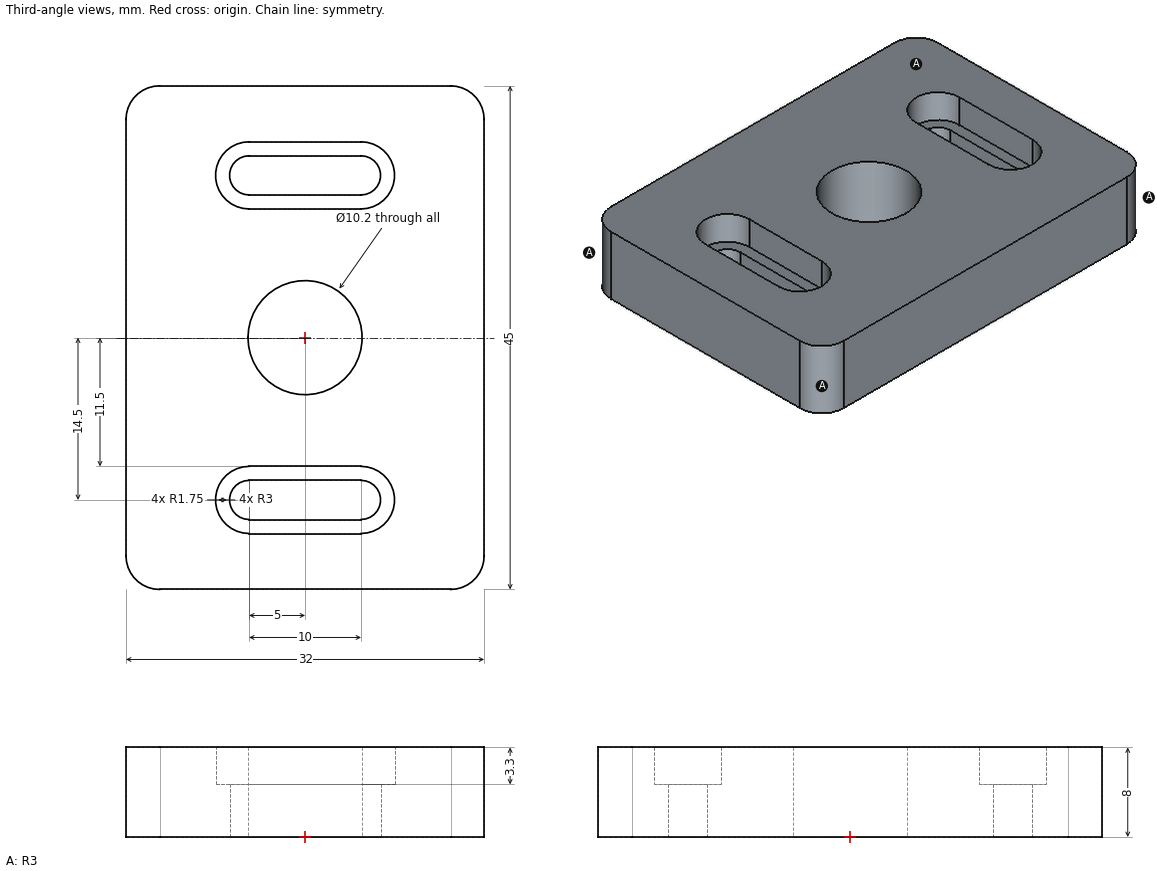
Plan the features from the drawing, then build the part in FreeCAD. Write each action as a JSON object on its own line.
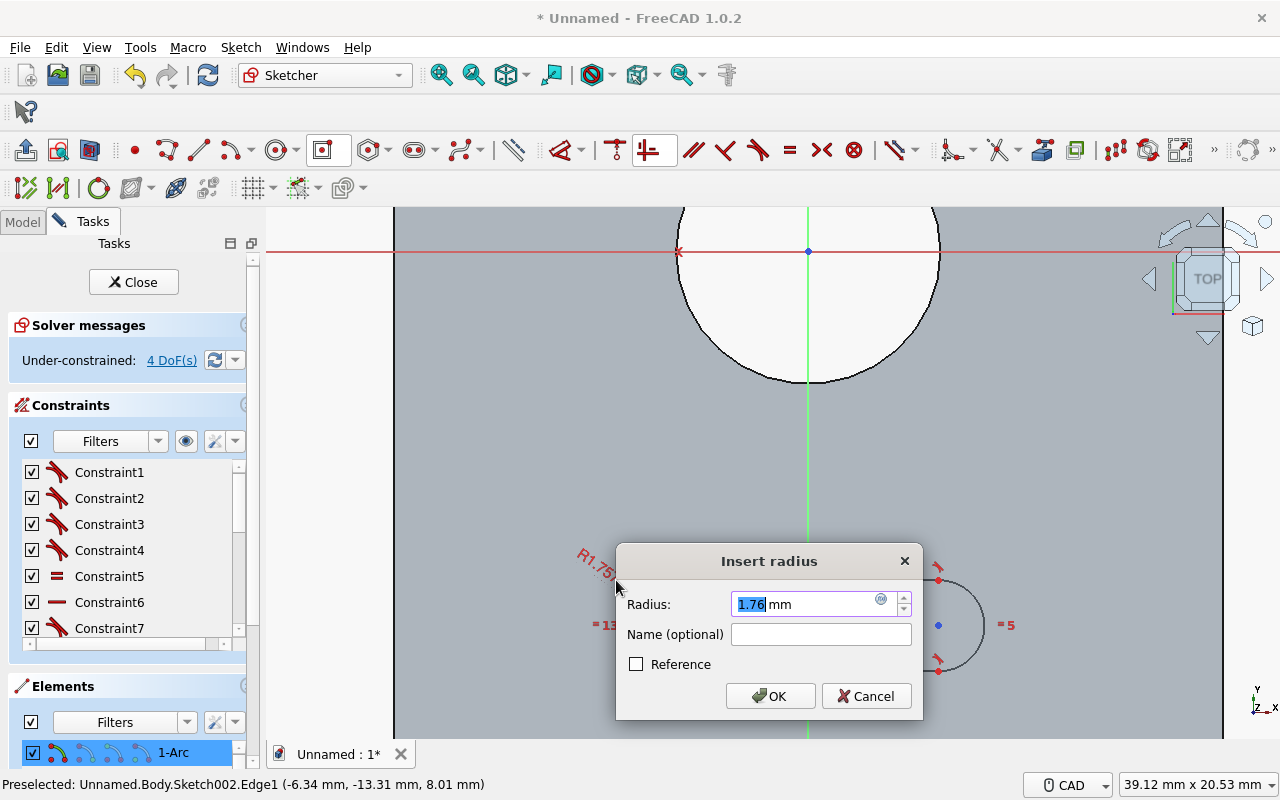
{"action": "type", "text": "1.75"}
{"action": "key", "text": "Return"}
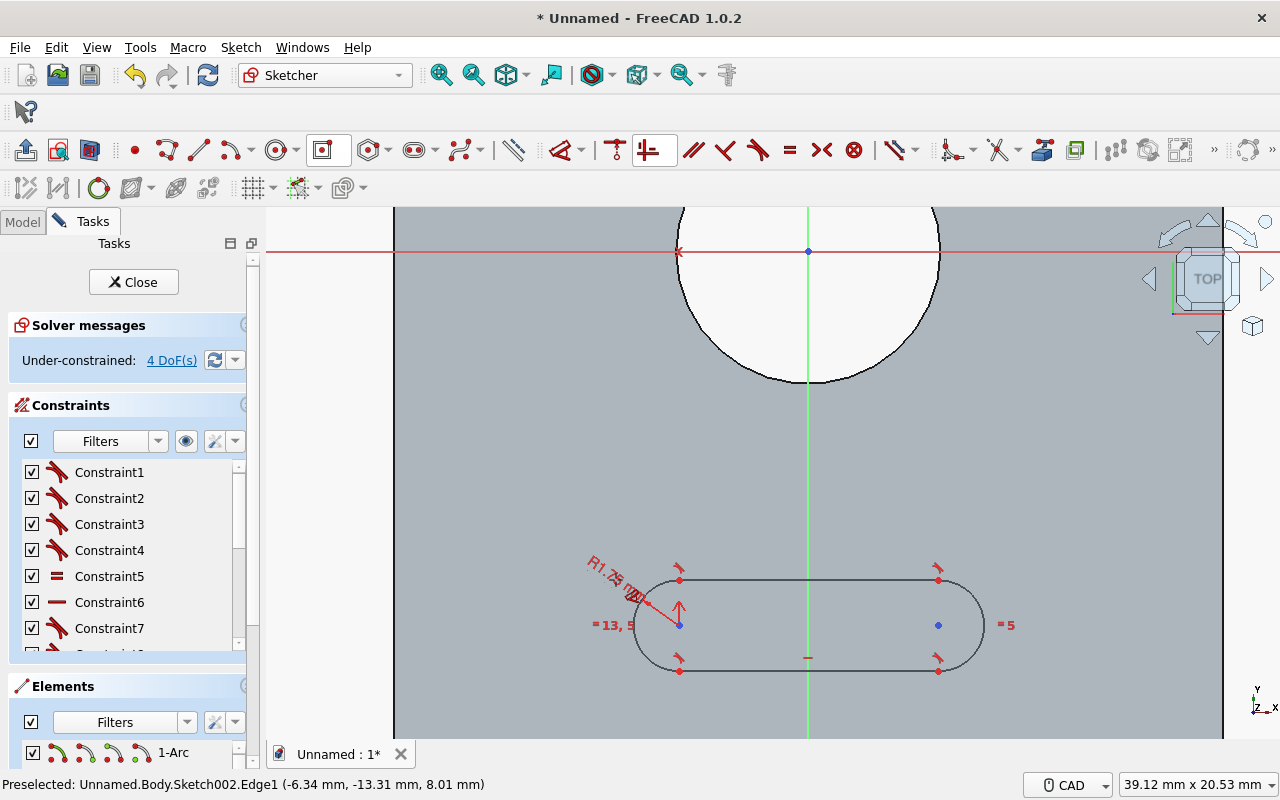
{"action": "left_click", "coordinate": [757, 580]}
{"action": "left_click", "coordinate": [749, 614]}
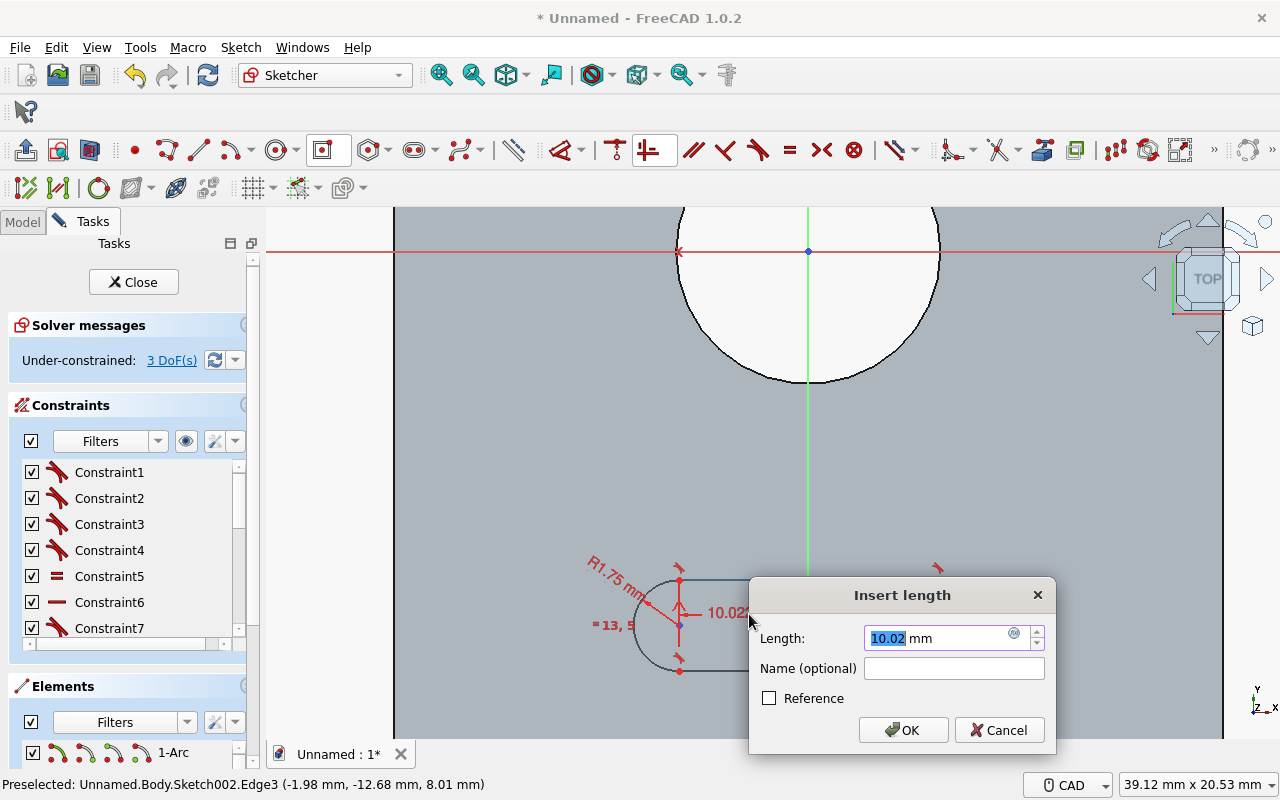
{"action": "type", "text": "10"}
{"action": "key", "text": "Return"}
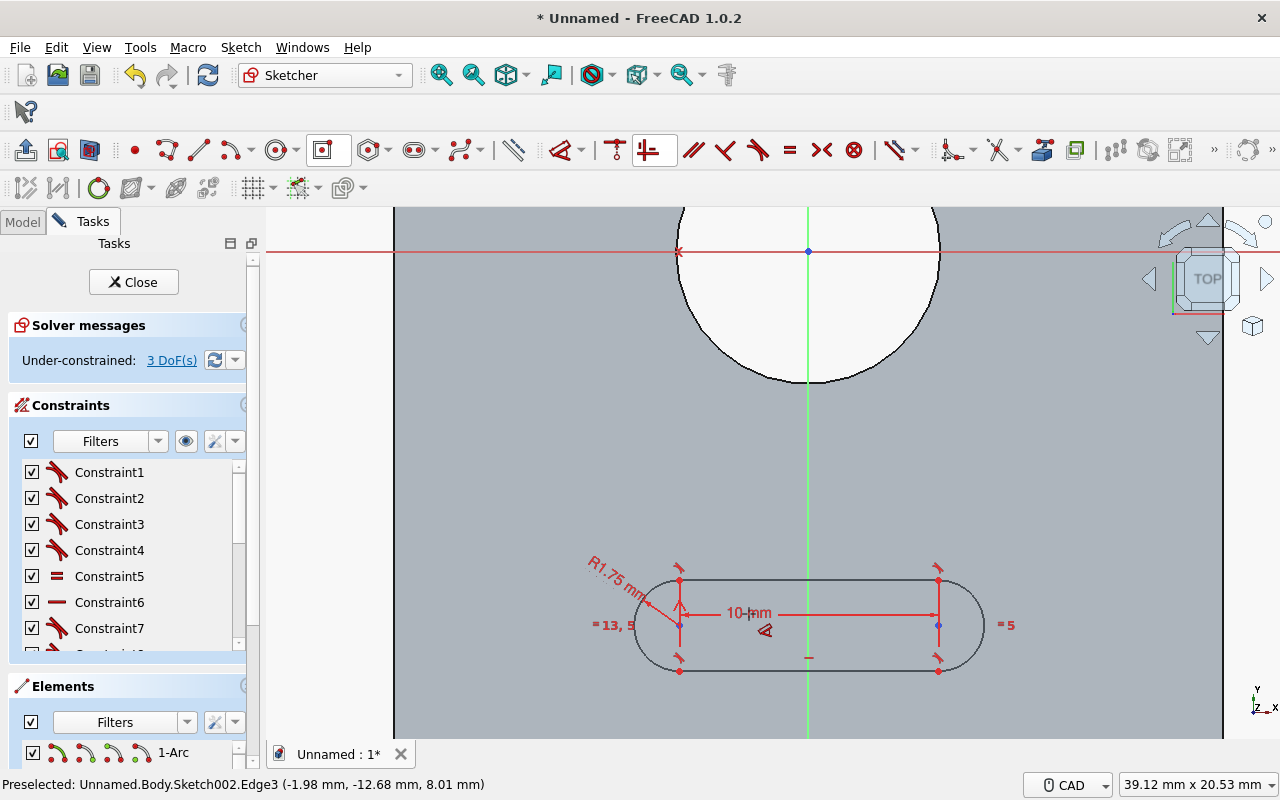
{"action": "scroll", "coordinate": [644, 602], "scroll_direction": "down", "scroll_amount": 5}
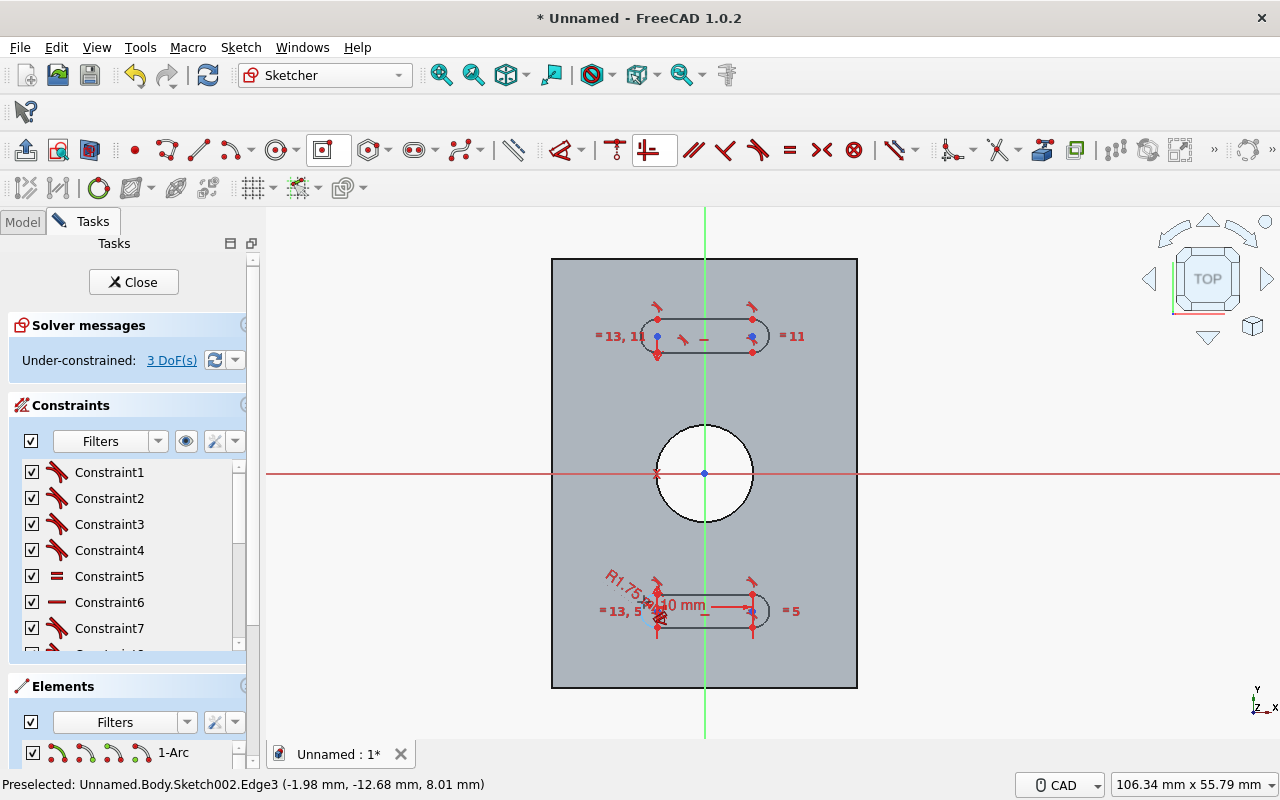
{"action": "left_click", "coordinate": [686, 319]}
{"action": "left_click", "coordinate": [683, 285]}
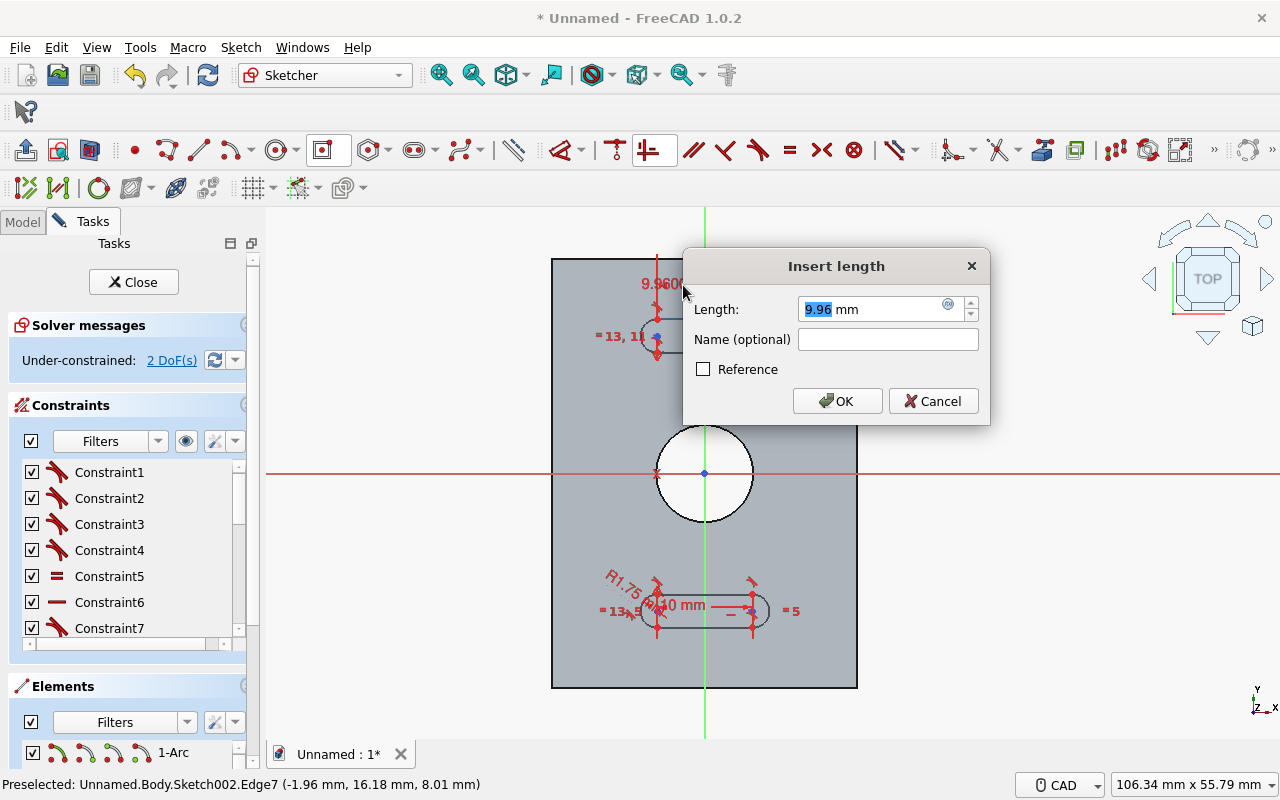
{"action": "type", "text": "10"}
{"action": "key", "text": "Return"}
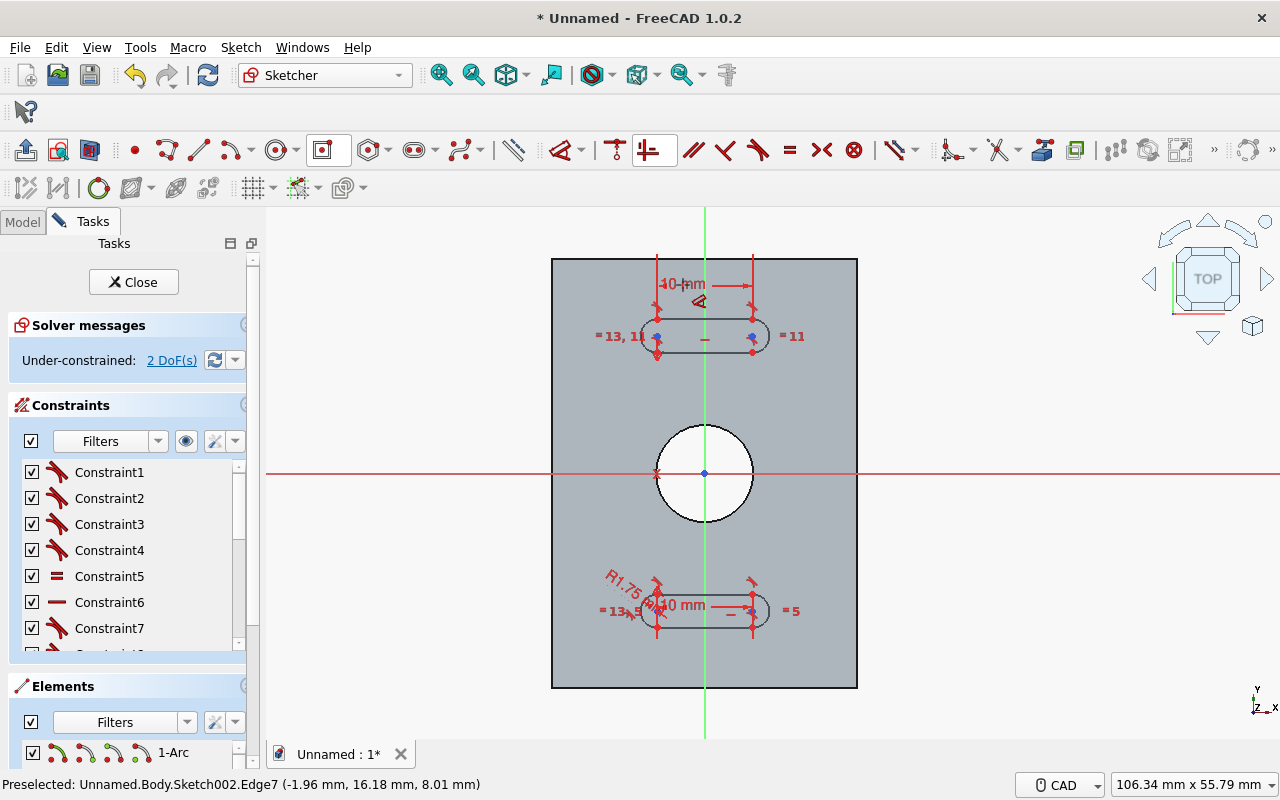
{"action": "left_click", "coordinate": [657, 595]}
{"action": "left_click", "coordinate": [681, 440]}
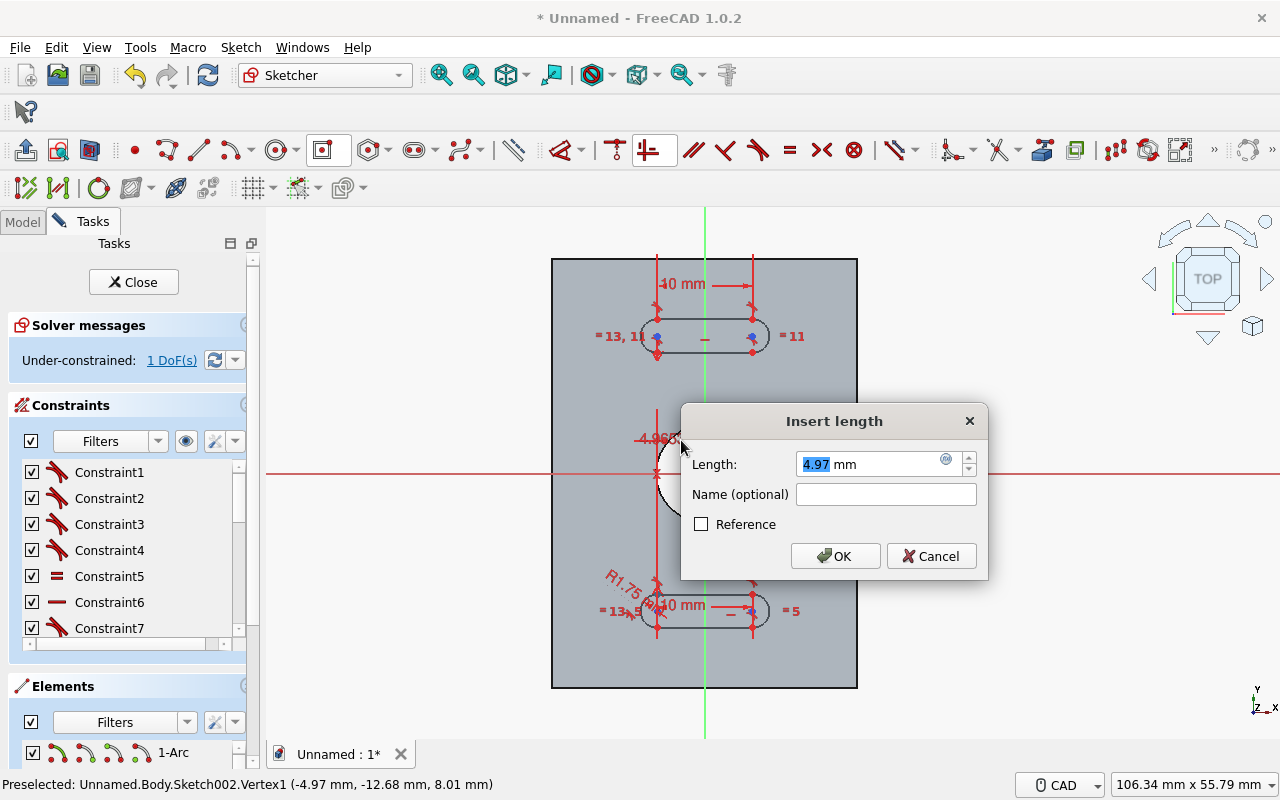
{"action": "type", "text": "5"}
{"action": "key", "text": "Return"}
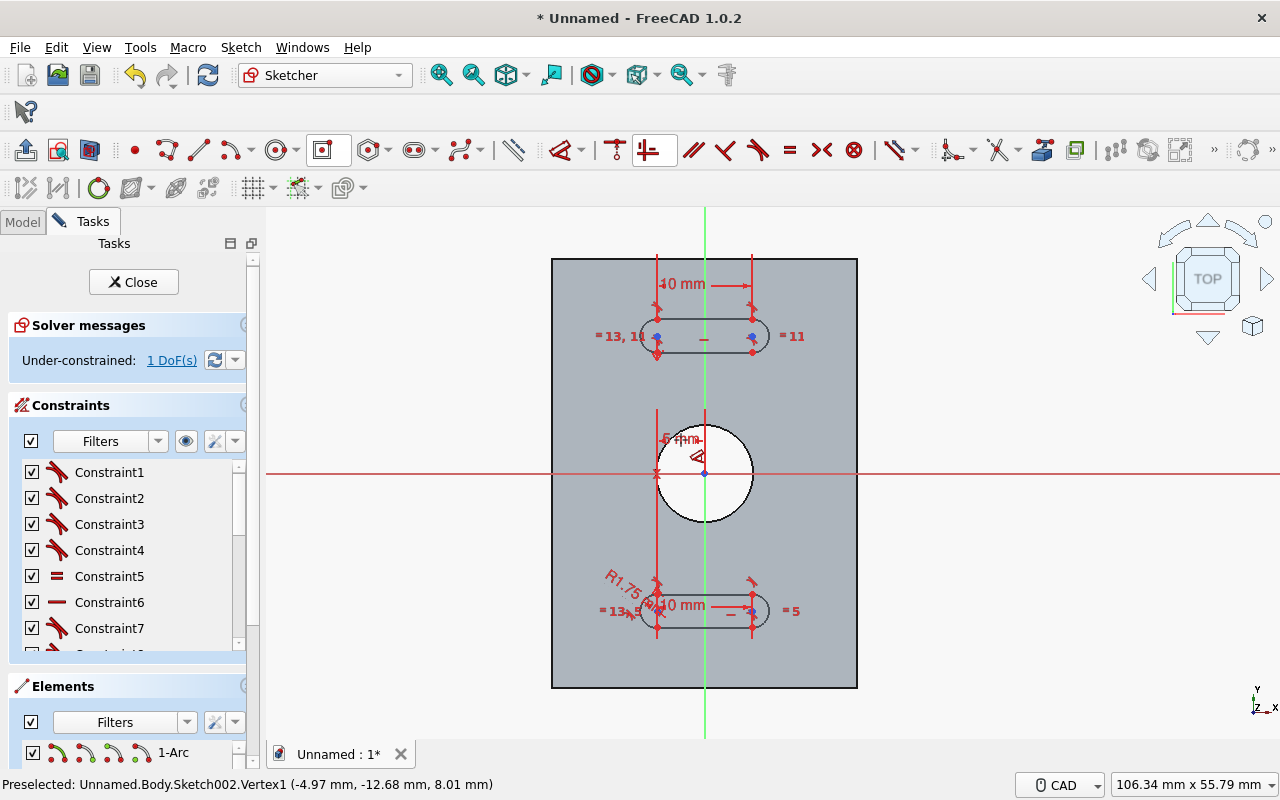
{"action": "left_click", "coordinate": [657, 611]}
{"action": "left_click", "coordinate": [623, 542]}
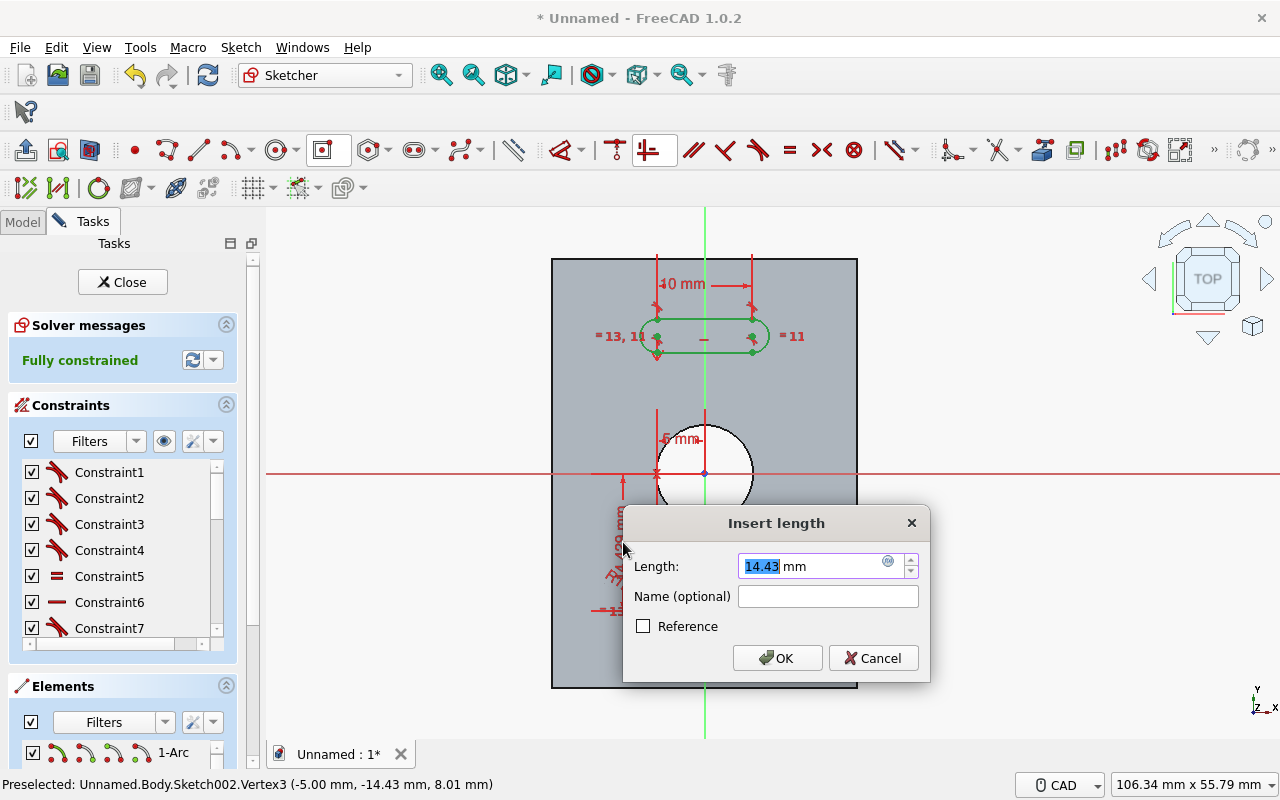
{"action": "type", "text": "14.5"}
{"action": "key", "text": "Return"}
{"action": "key", "text": "Escape"}